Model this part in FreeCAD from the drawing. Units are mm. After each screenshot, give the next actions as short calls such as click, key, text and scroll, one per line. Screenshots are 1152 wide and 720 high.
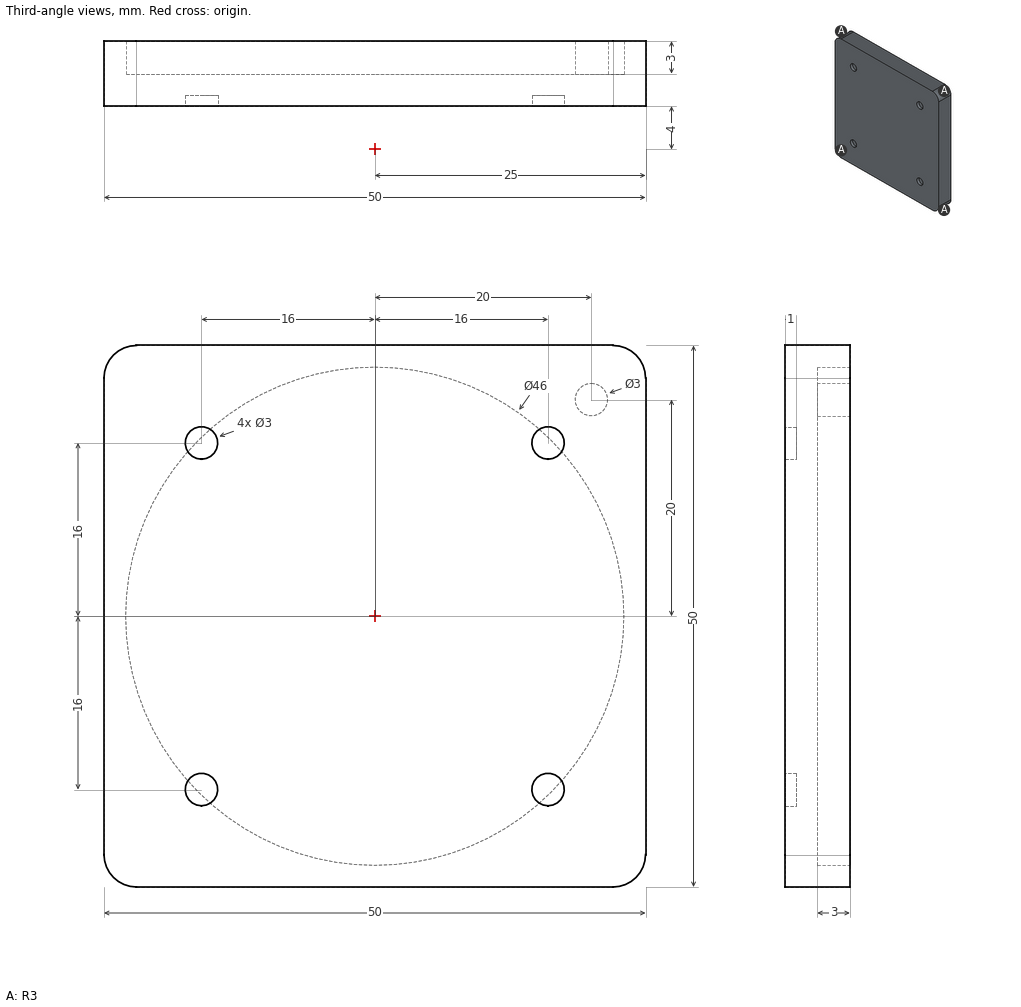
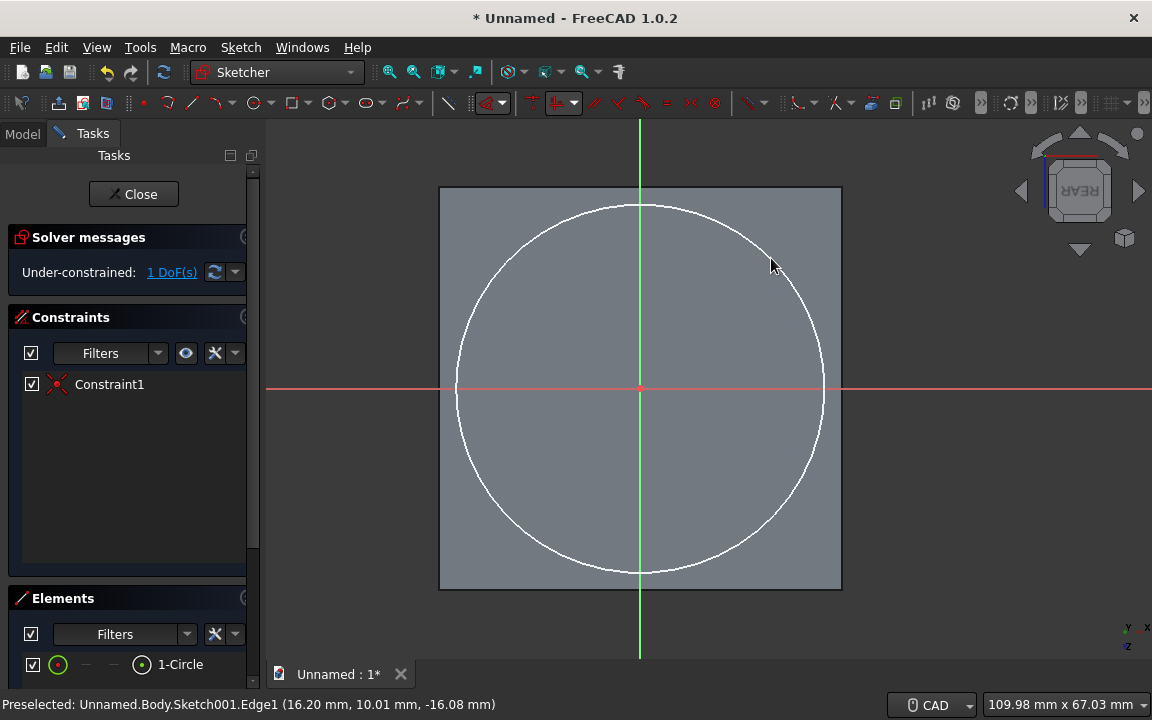
click(770, 258)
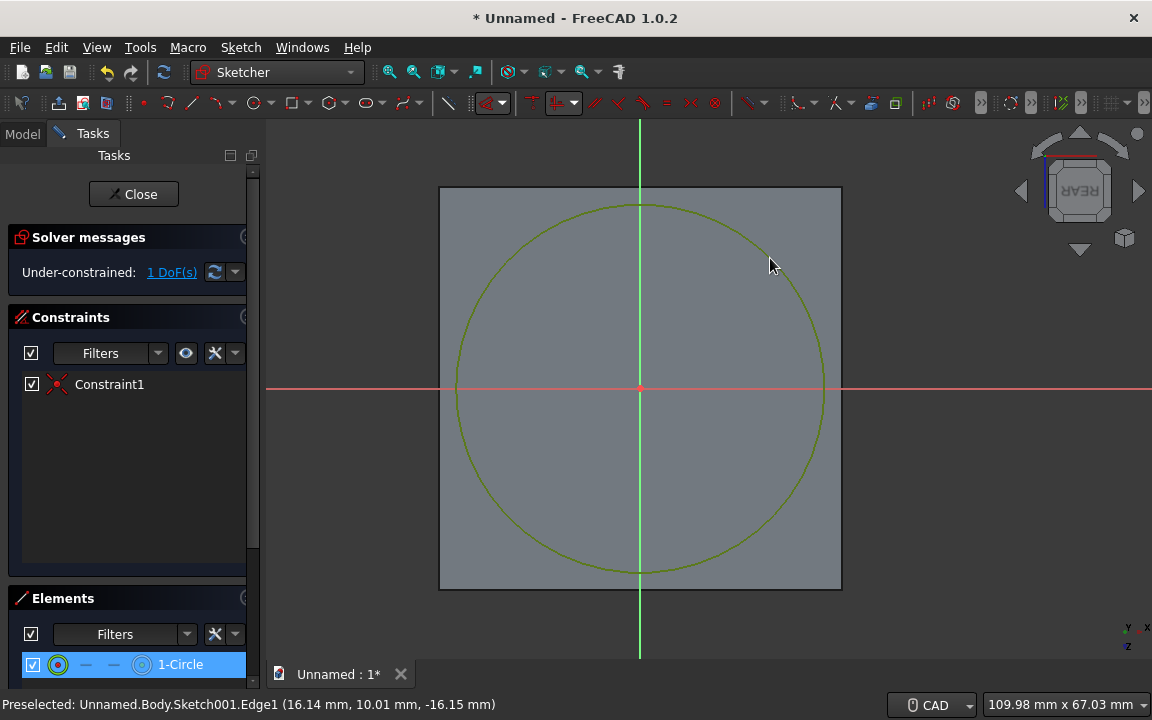
click(504, 104)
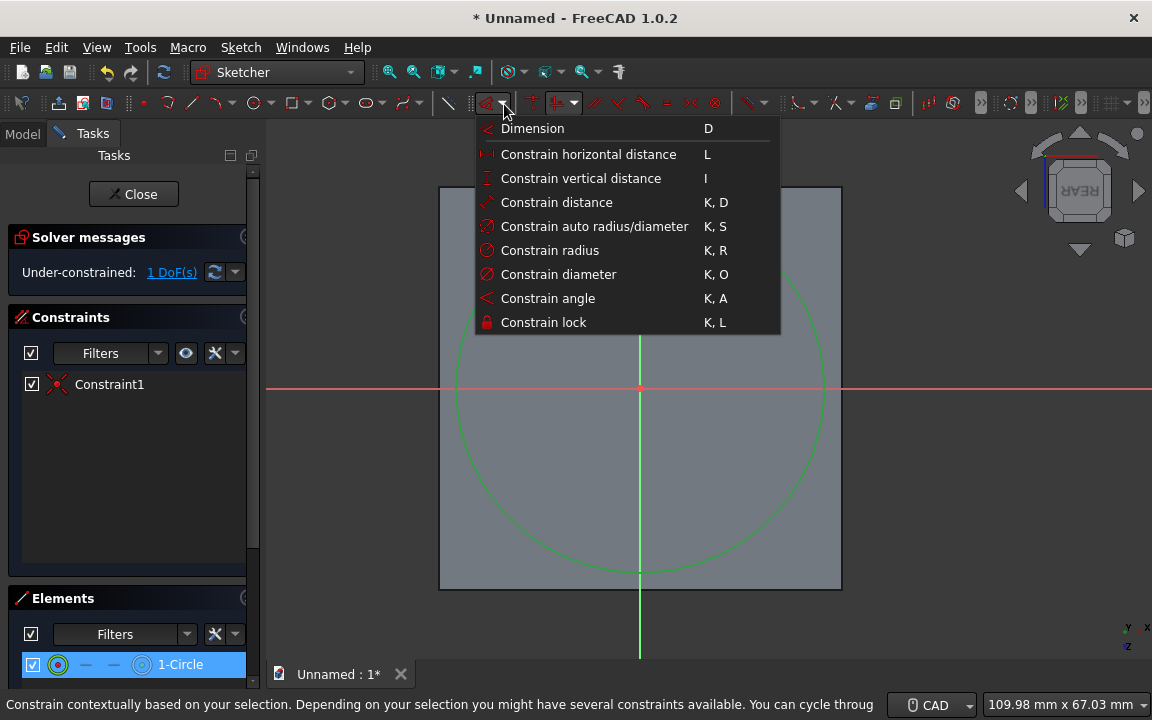
click(628, 274)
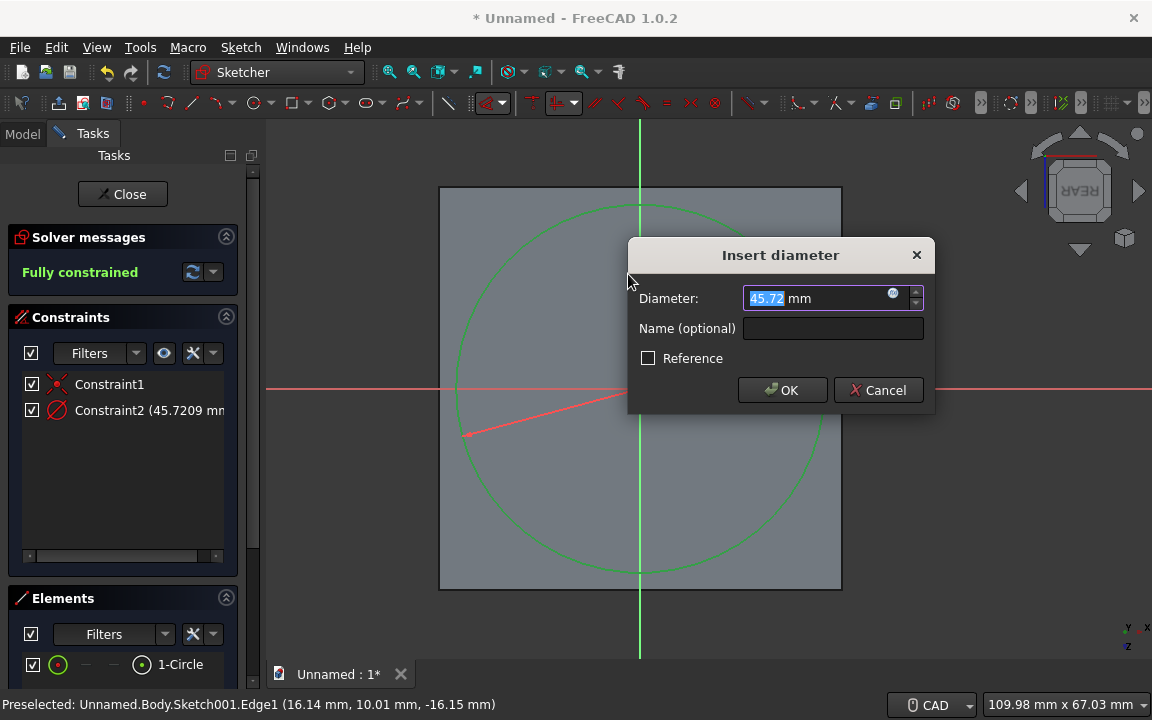
text(46)
key(Return)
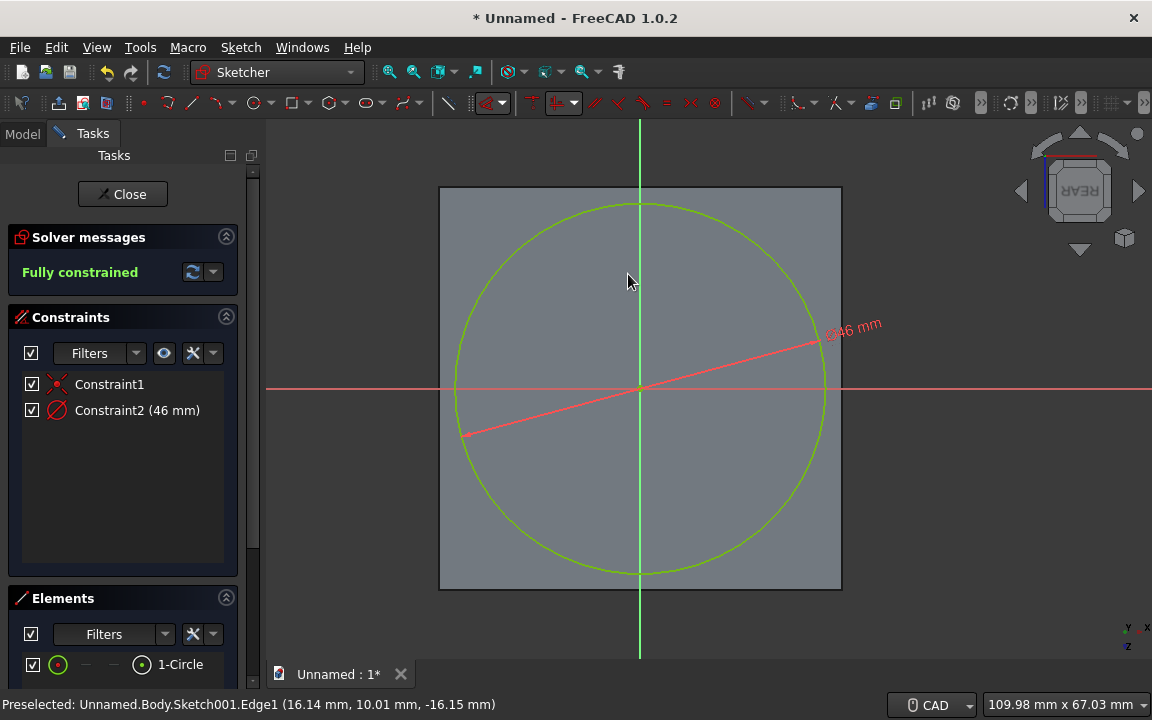
click(123, 194)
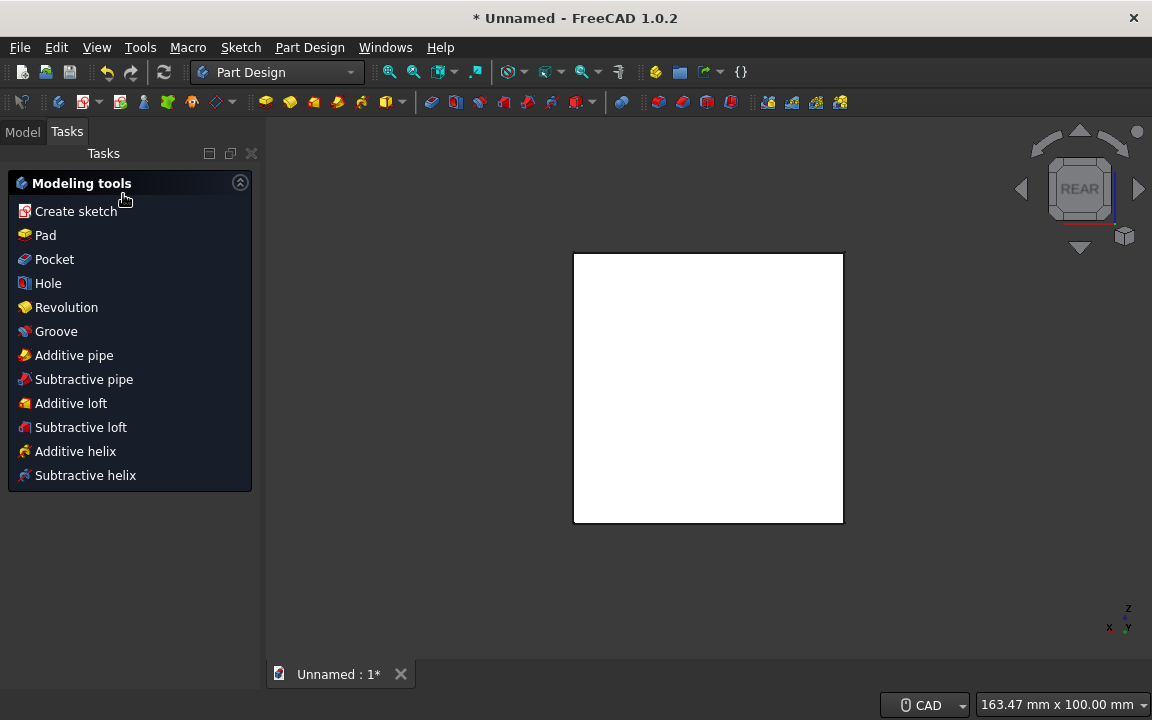
click(432, 102)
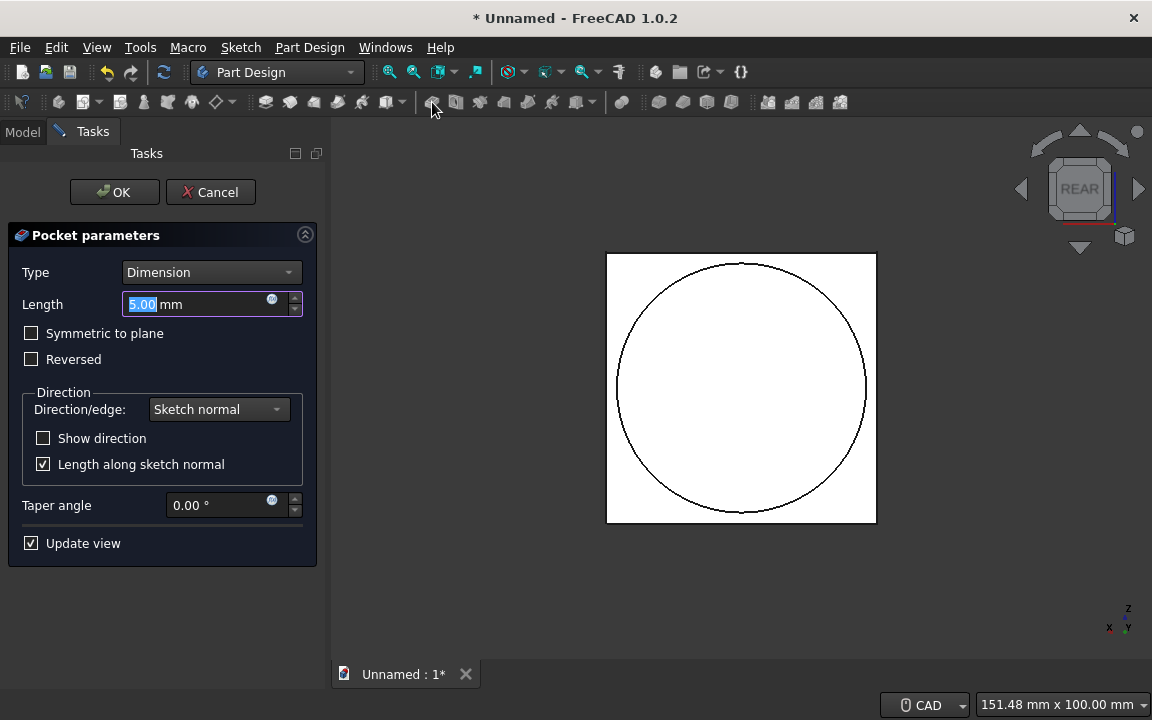
text(3)
key(Tab)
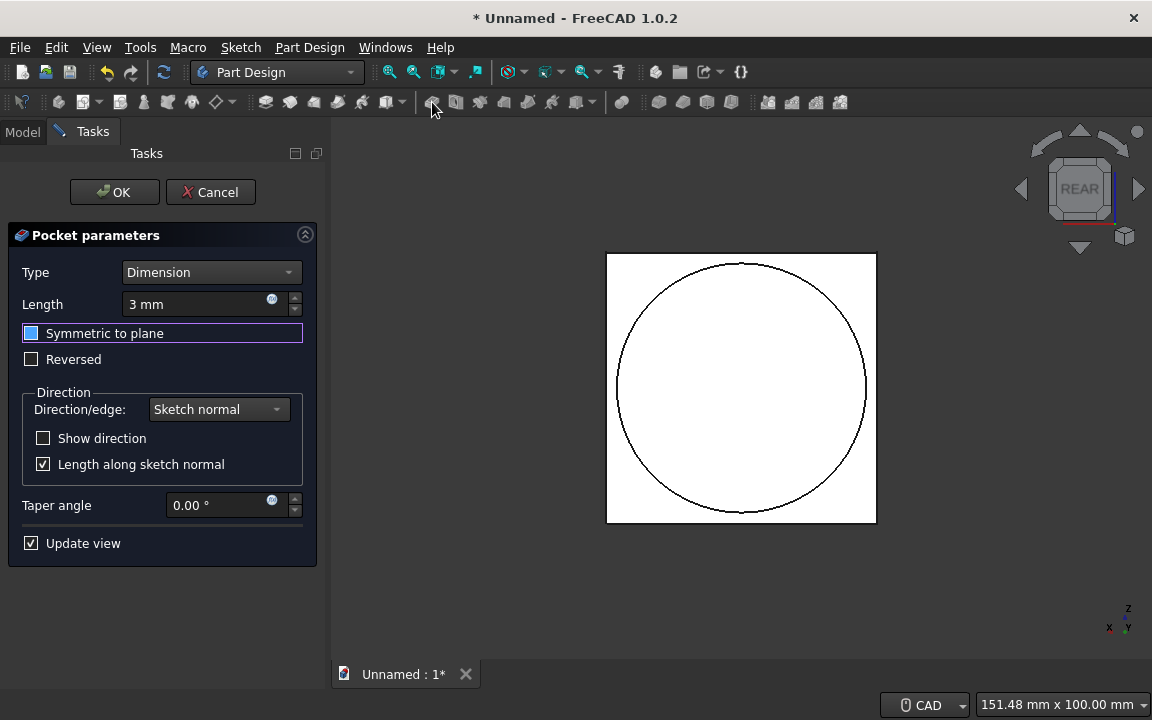
click(115, 192)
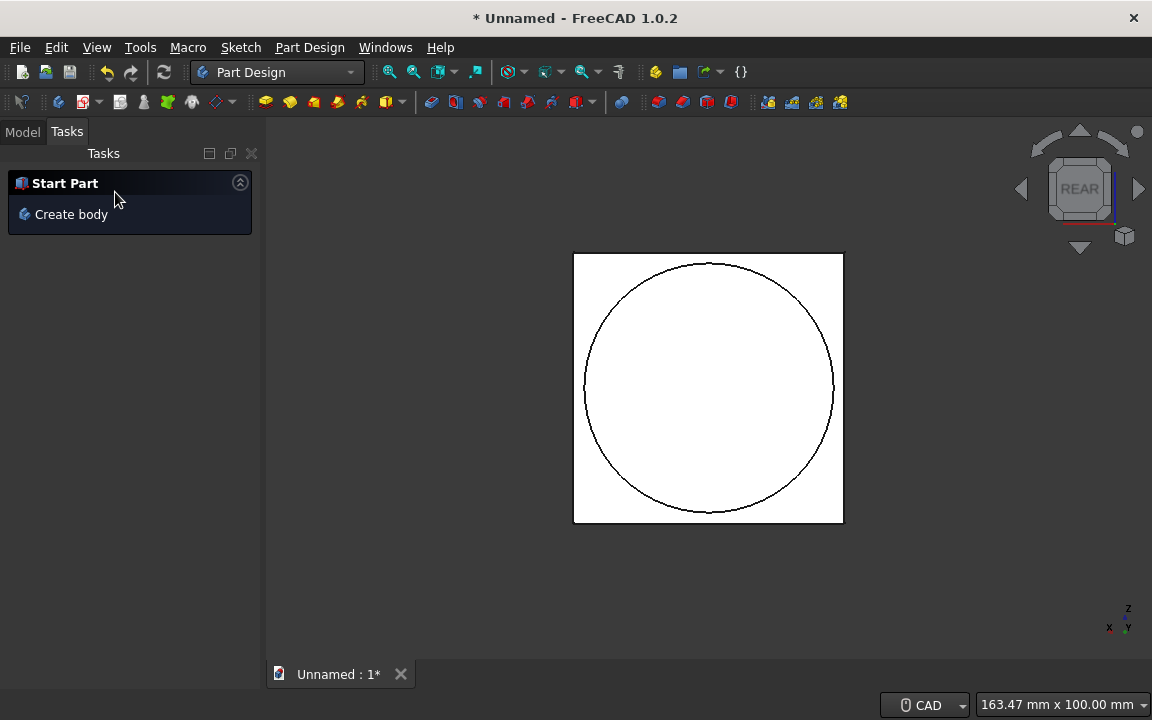
click(825, 503)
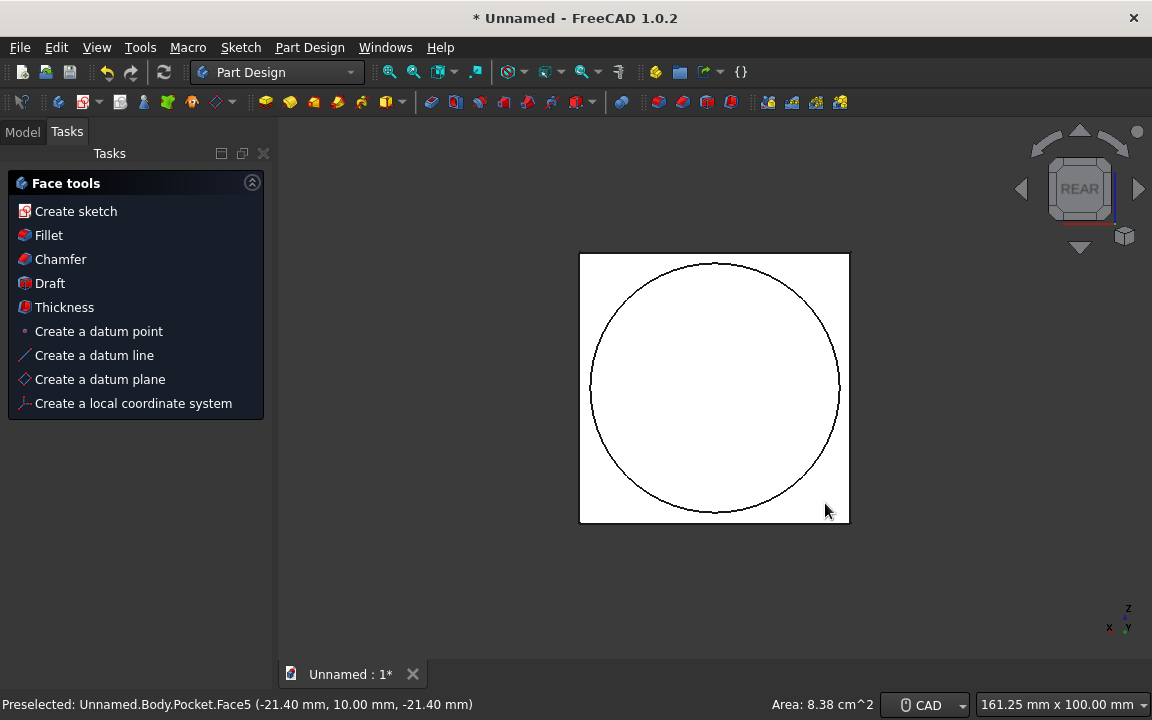
click(84, 102)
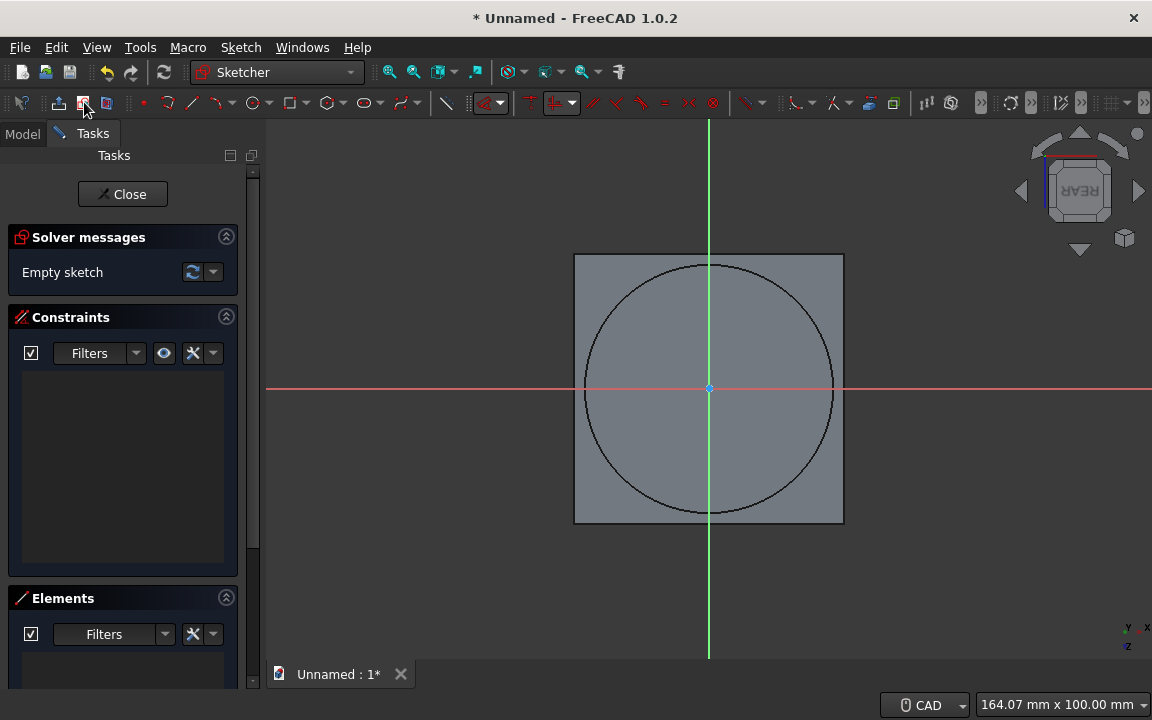
scroll(826, 503, up, 15)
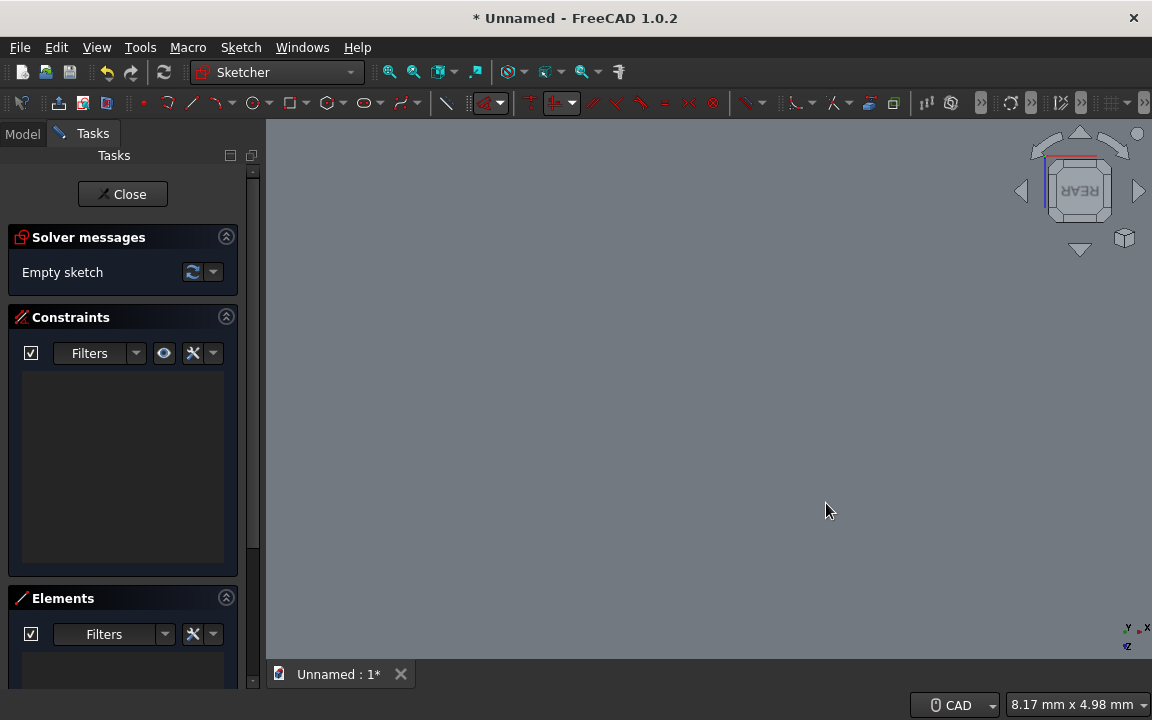
click(254, 104)